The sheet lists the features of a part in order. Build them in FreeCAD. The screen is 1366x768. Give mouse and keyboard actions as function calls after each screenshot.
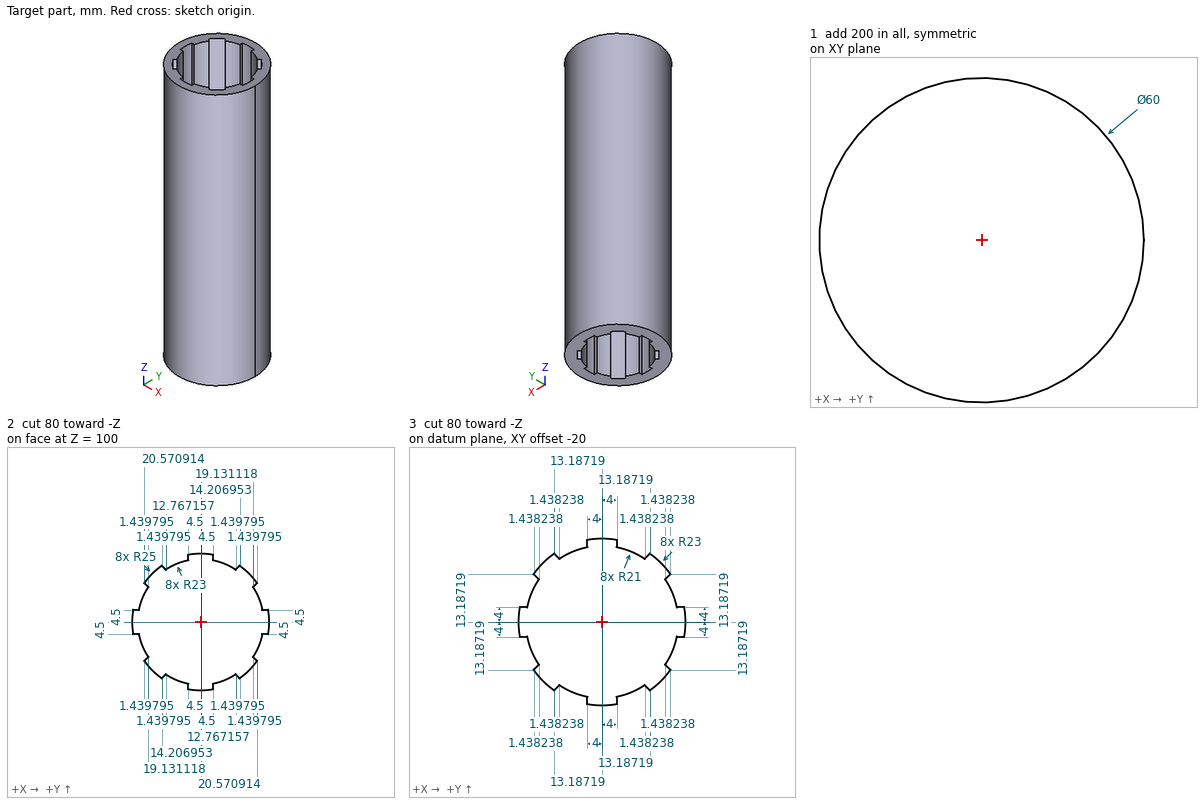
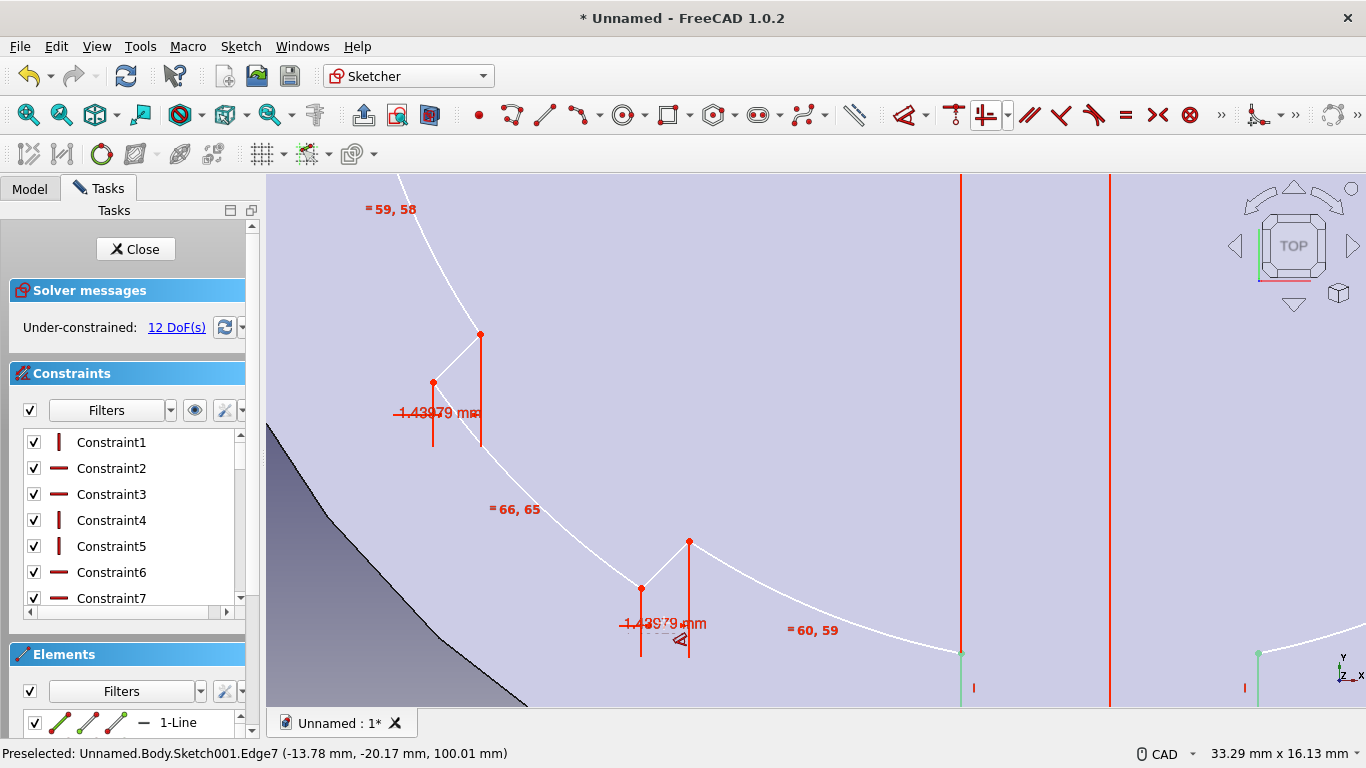
scroll(656, 575, down, 8)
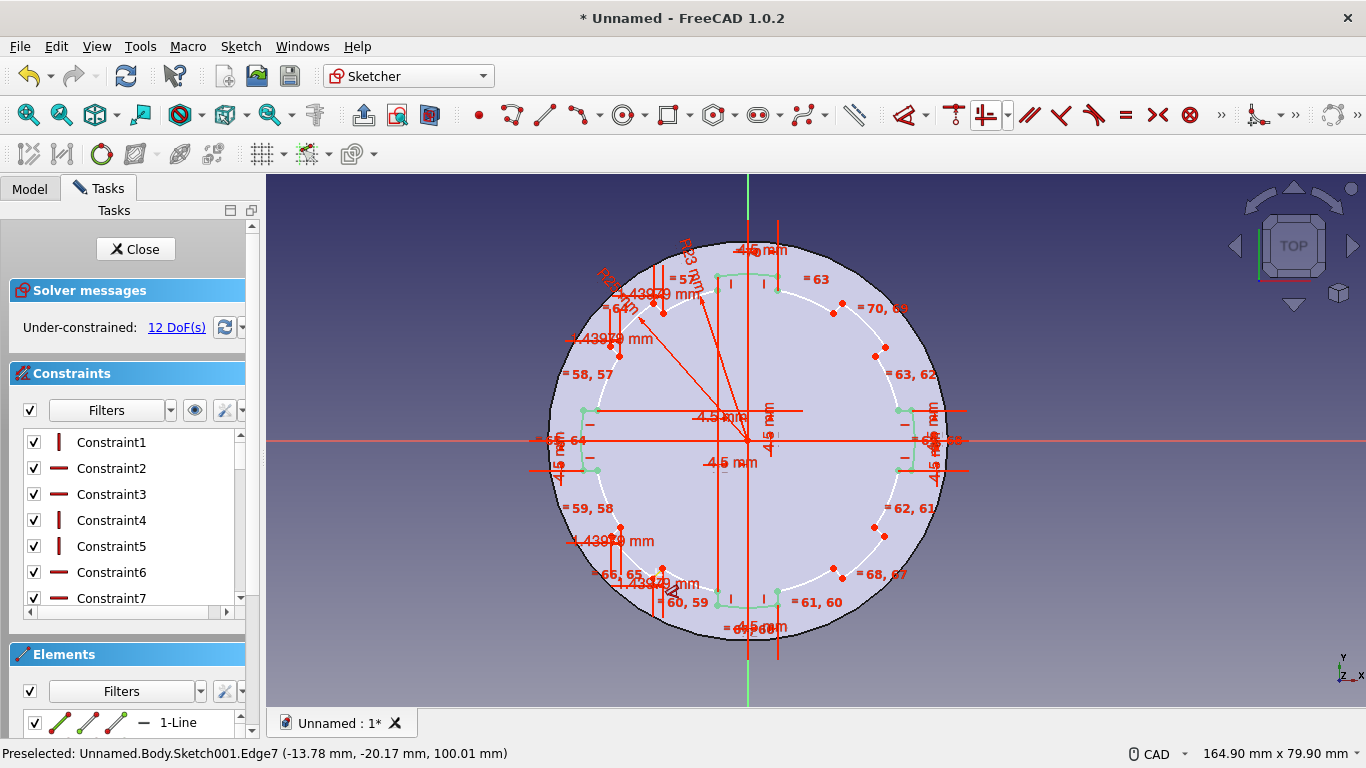
scroll(836, 571, up, 8)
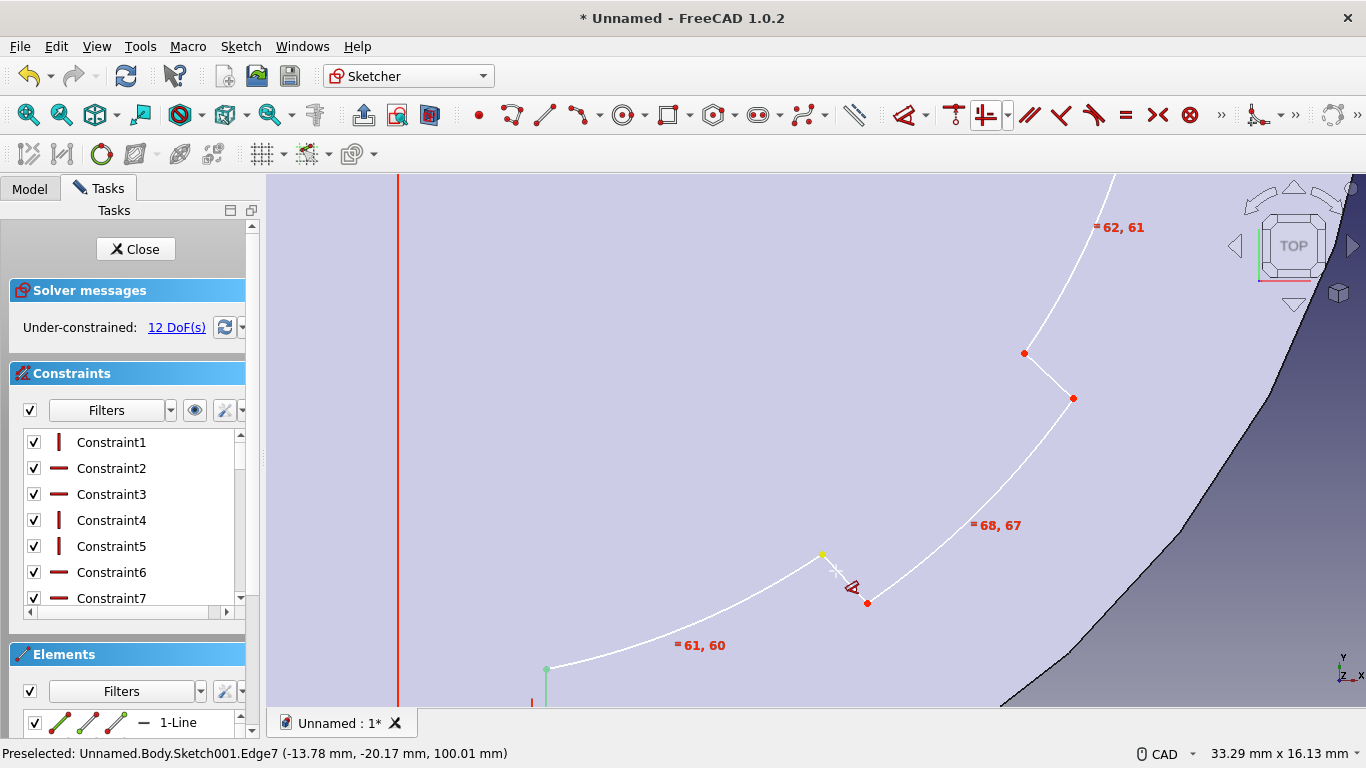
click(836, 569)
click(845, 637)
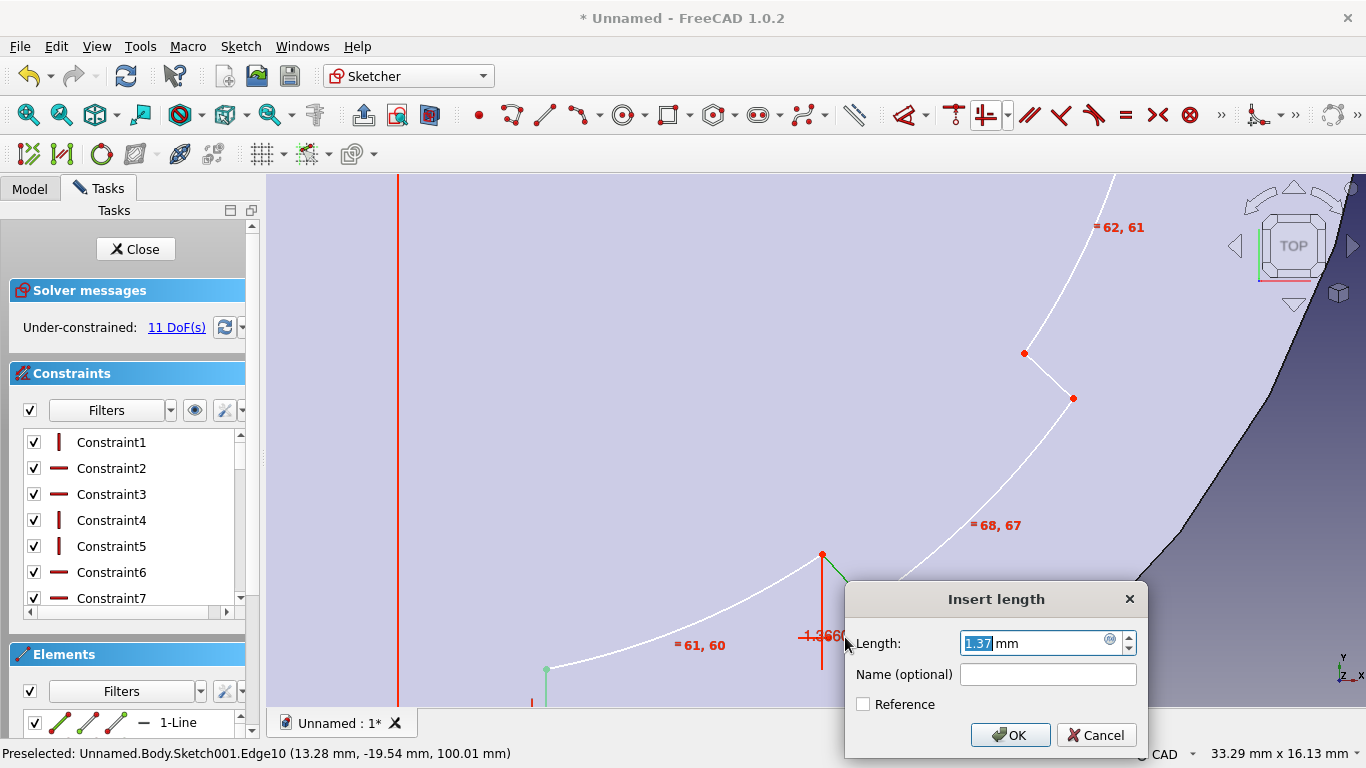
text(1.439795)
key(Return)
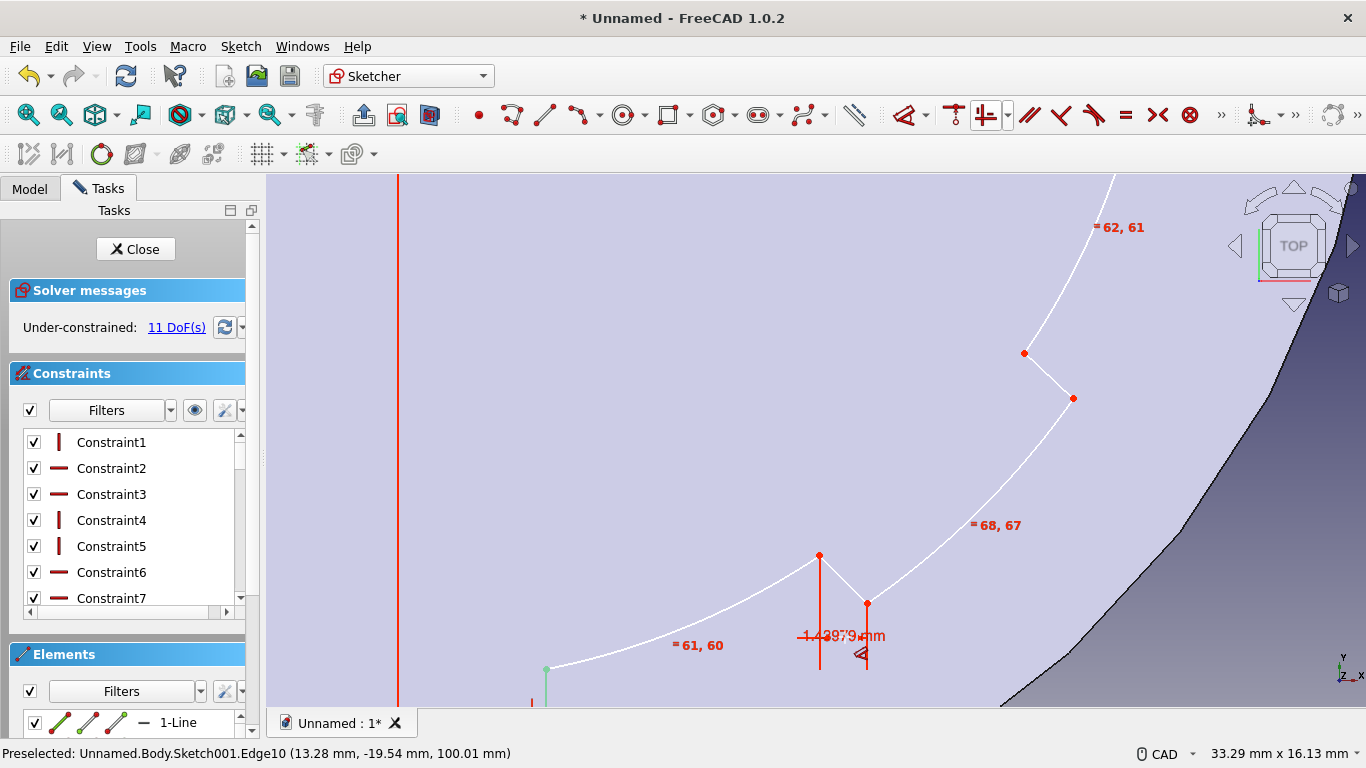
click(1059, 385)
click(1066, 433)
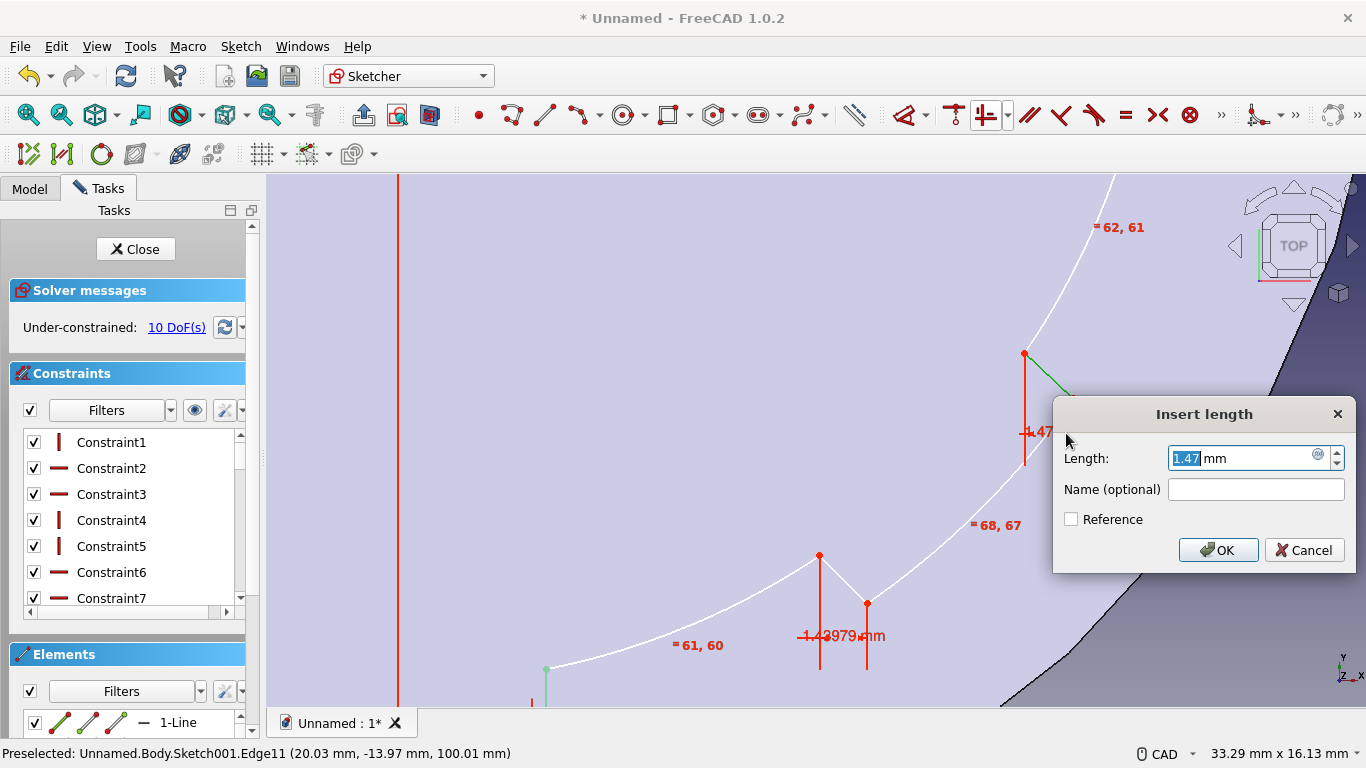
text(1.439795)
key(Return)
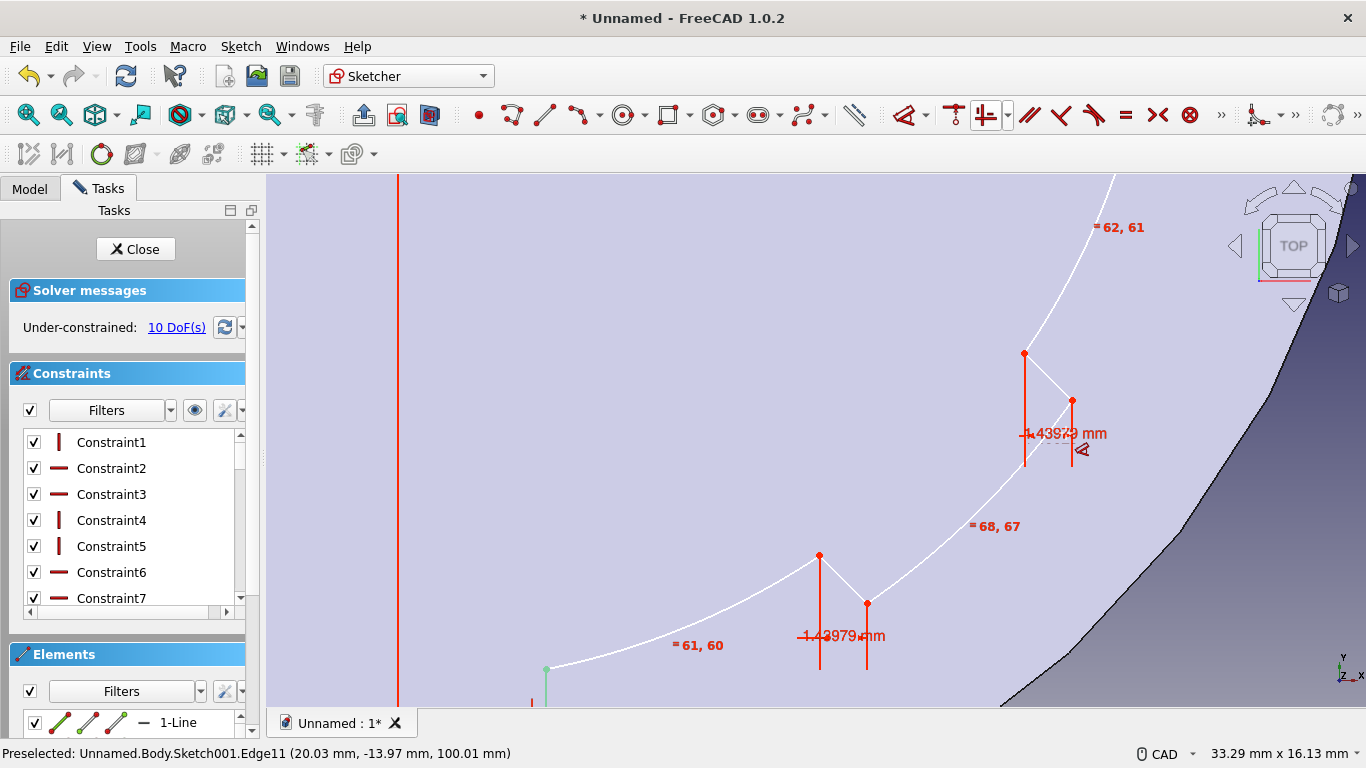
scroll(836, 571, down, 8)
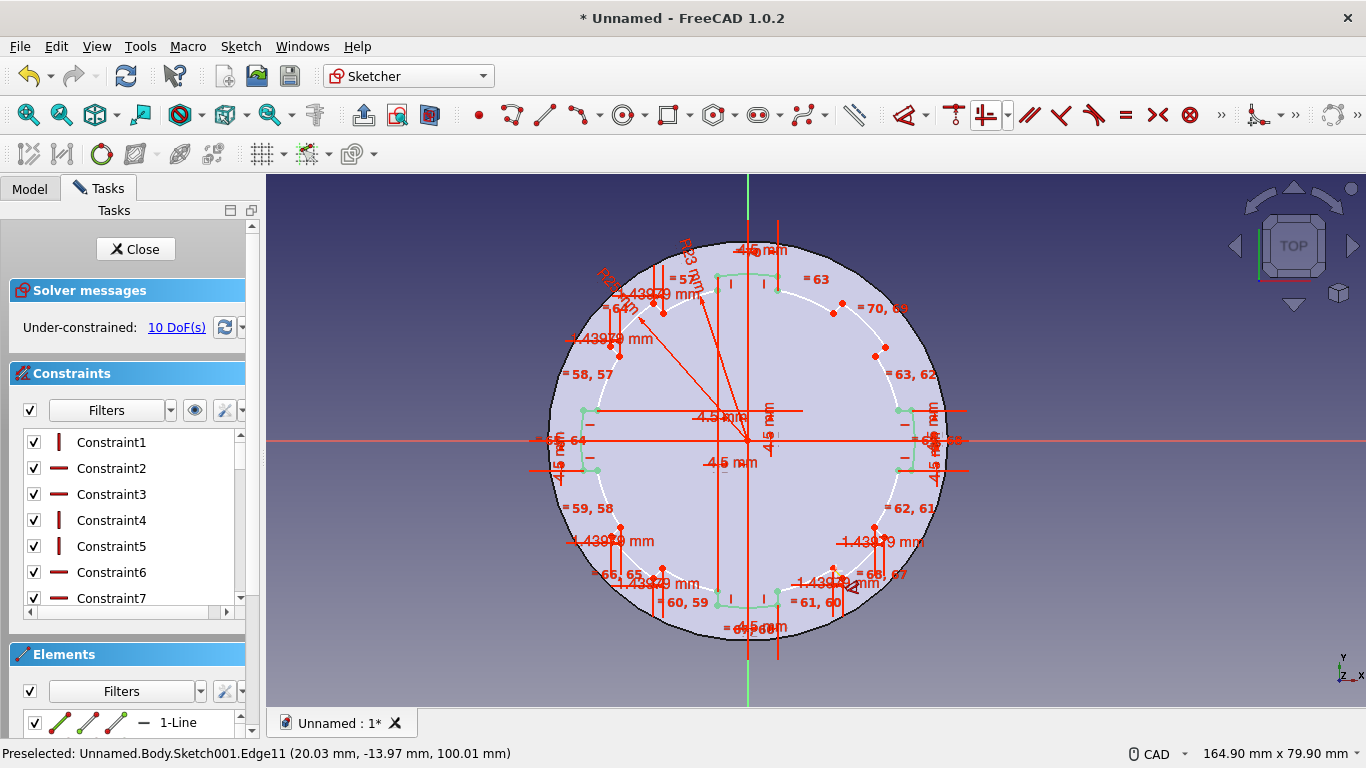
scroll(879, 354, up, 8)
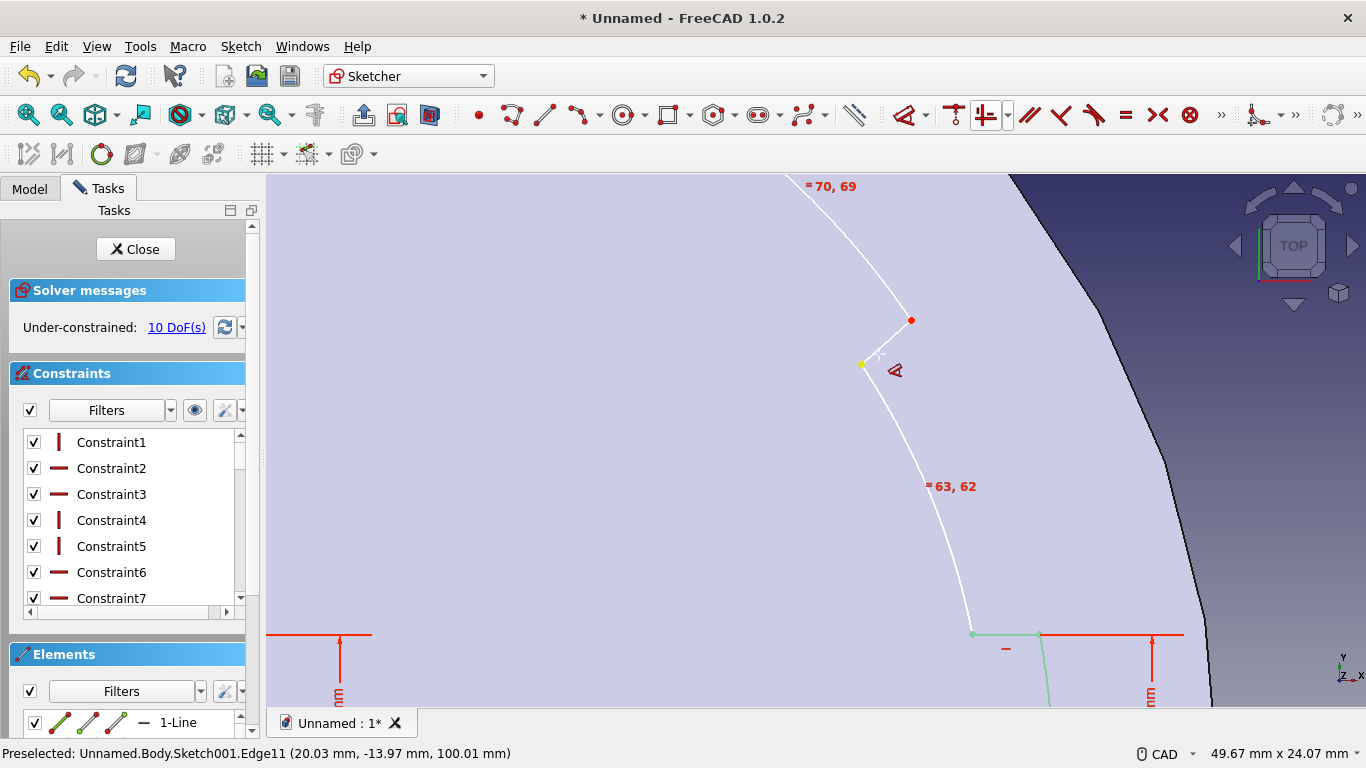
click(876, 351)
click(869, 286)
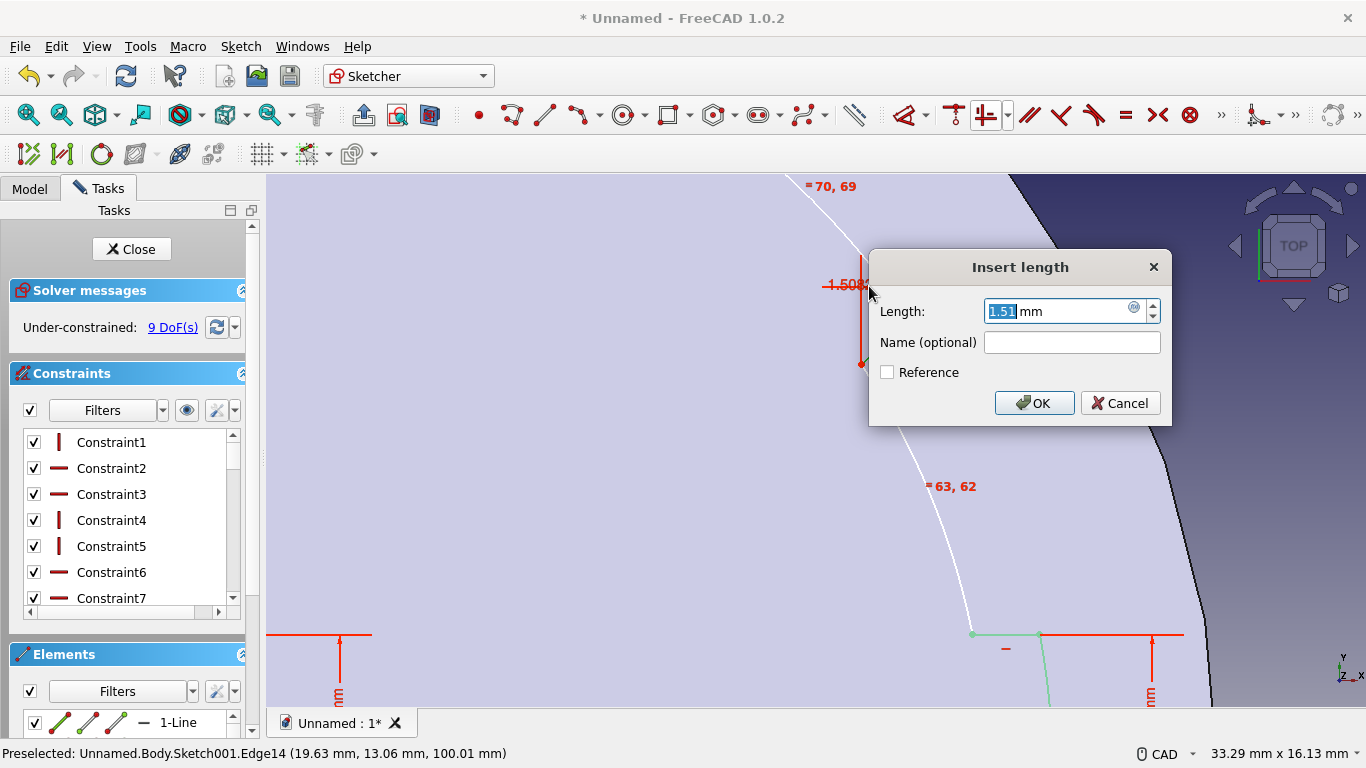
text(1.439795)
key(Return)